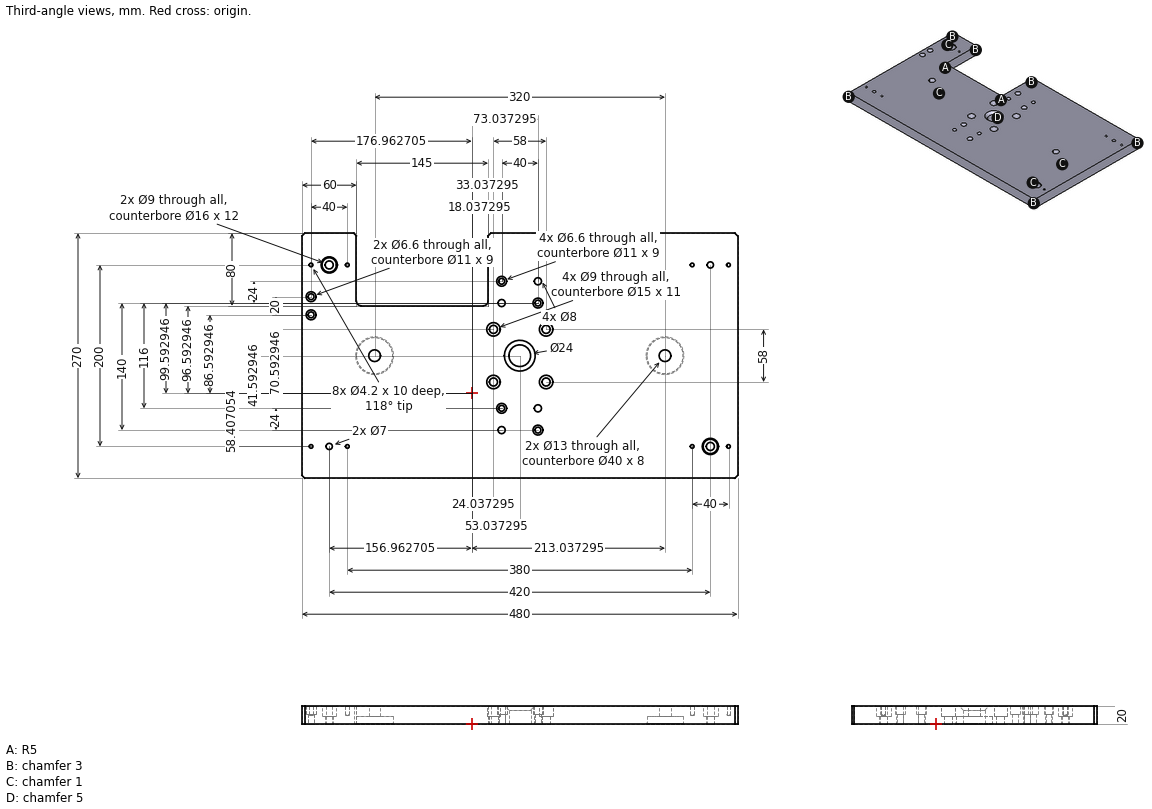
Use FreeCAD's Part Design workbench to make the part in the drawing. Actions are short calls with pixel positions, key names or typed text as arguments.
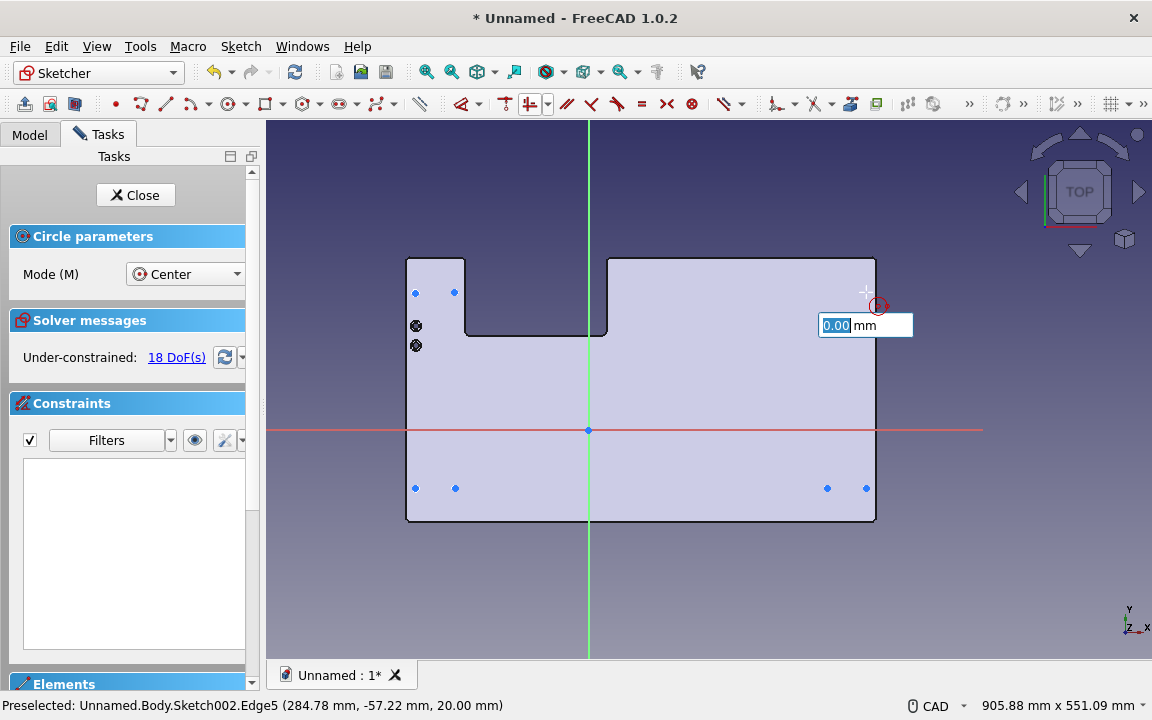
scroll(867, 290, up, 11)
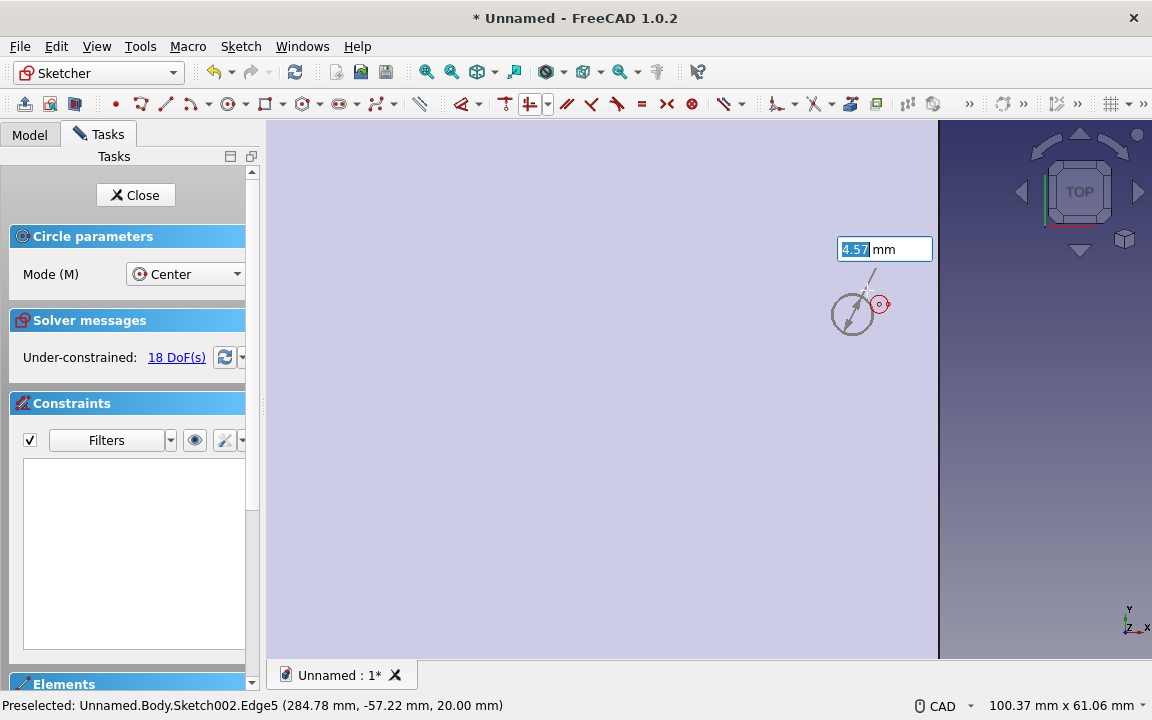
click(864, 290)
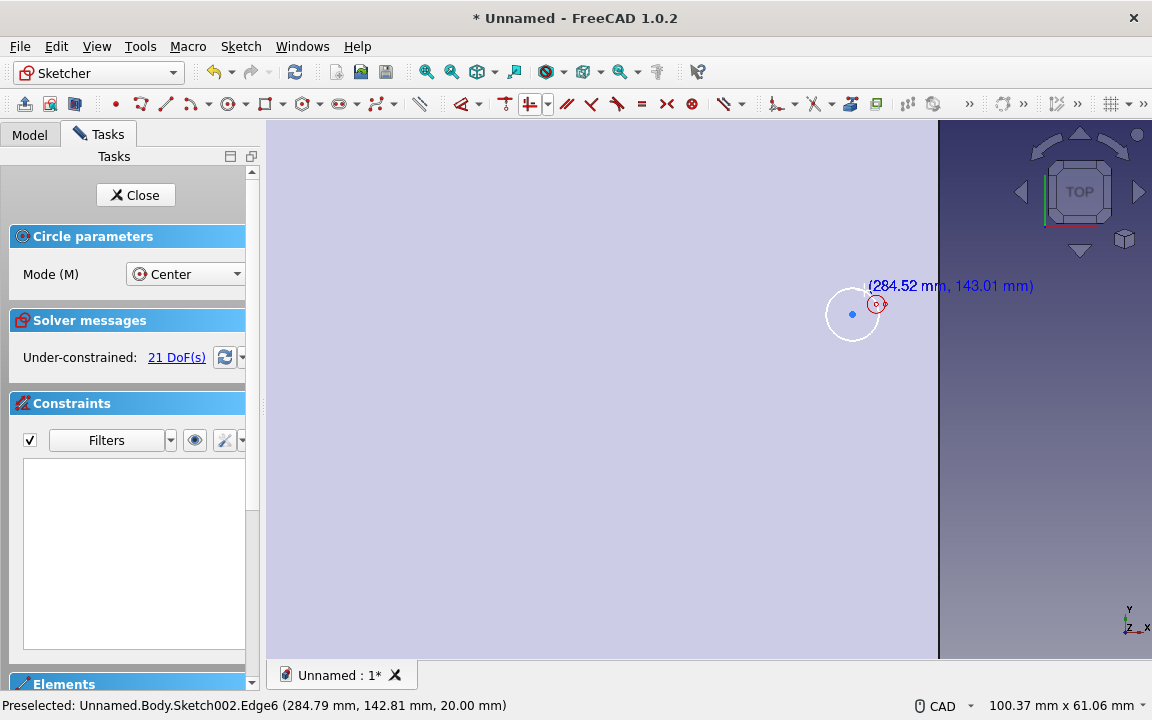
scroll(498, 304, up, 2)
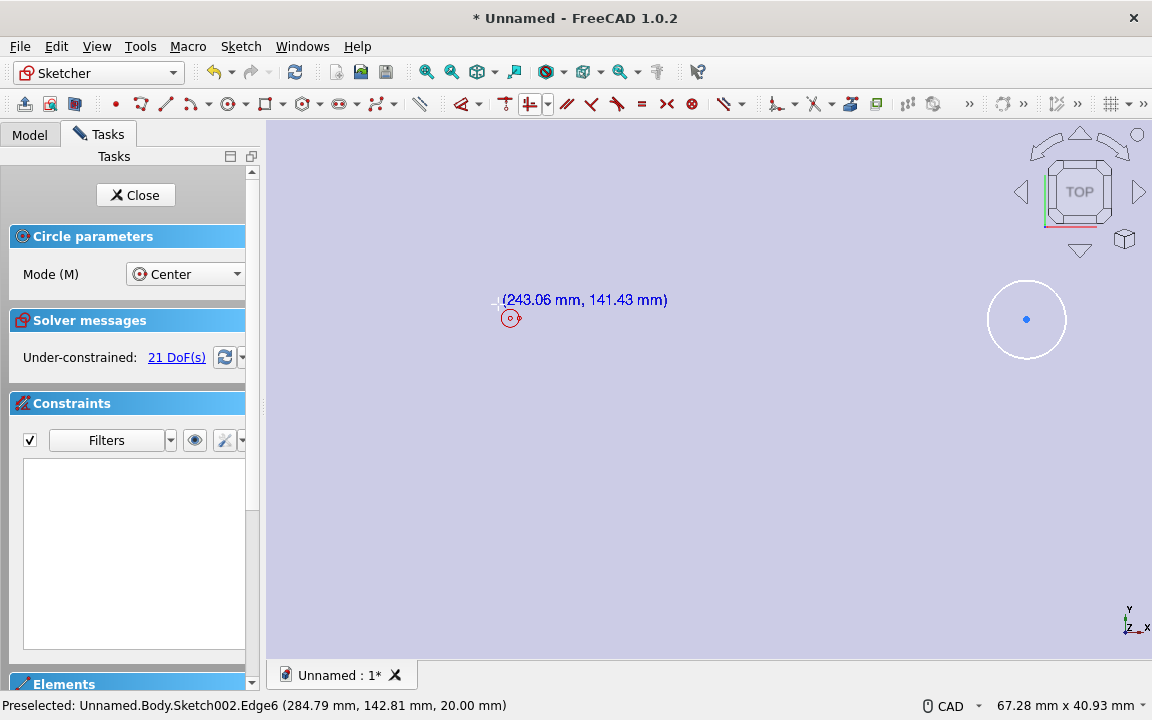
scroll(853, 291, down, 13)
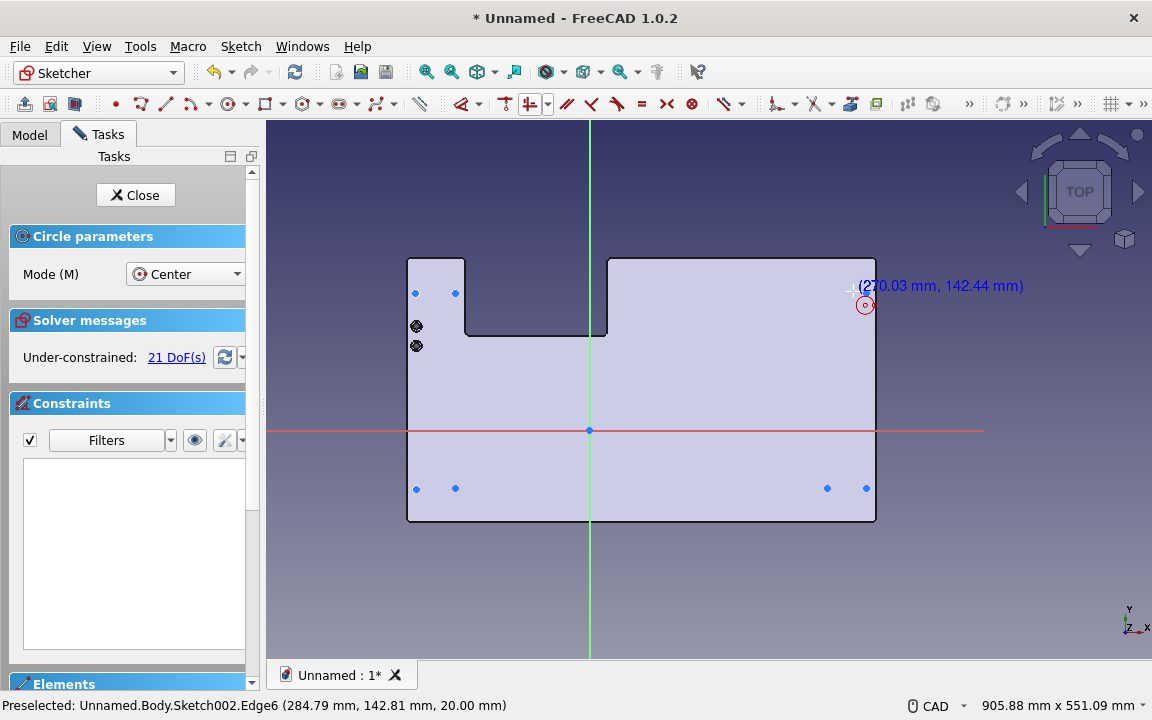
click(827, 292)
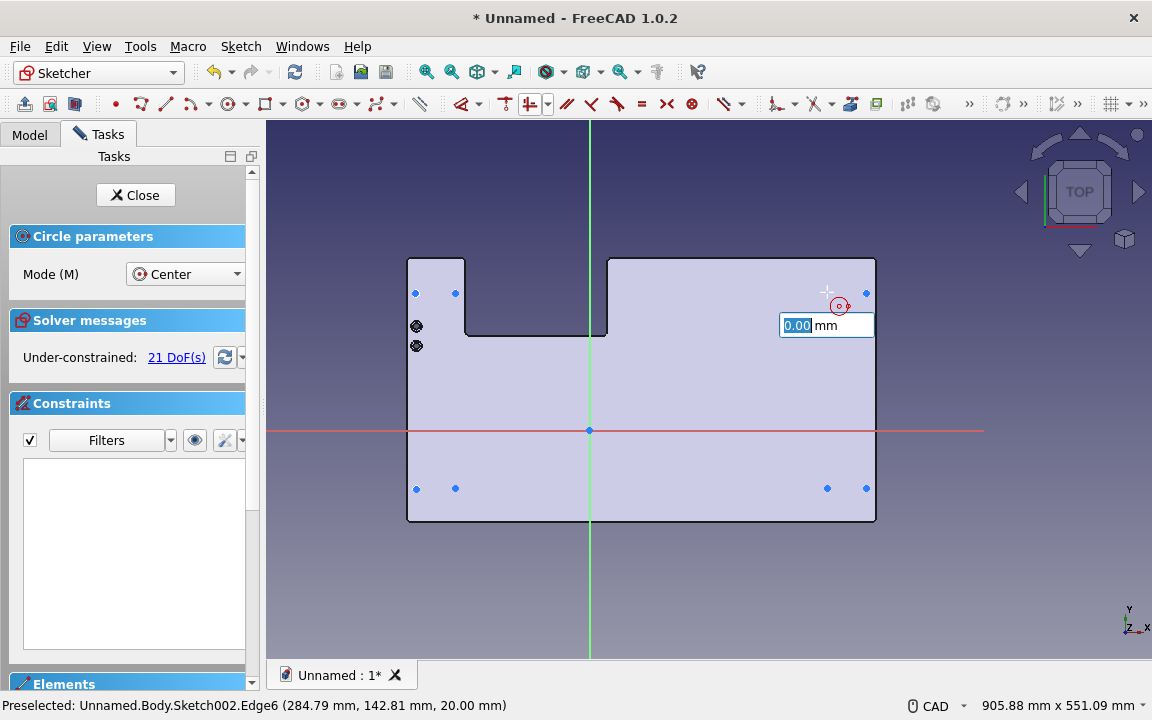
scroll(829, 291, up, 11)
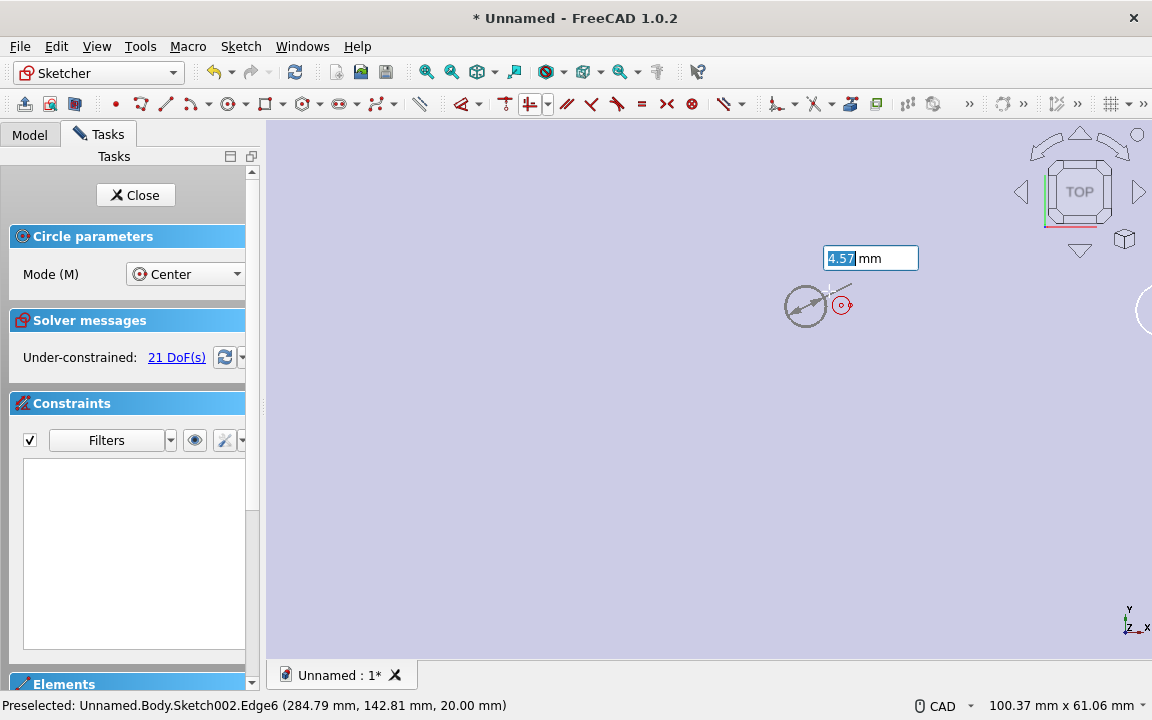
click(821, 286)
key(Escape)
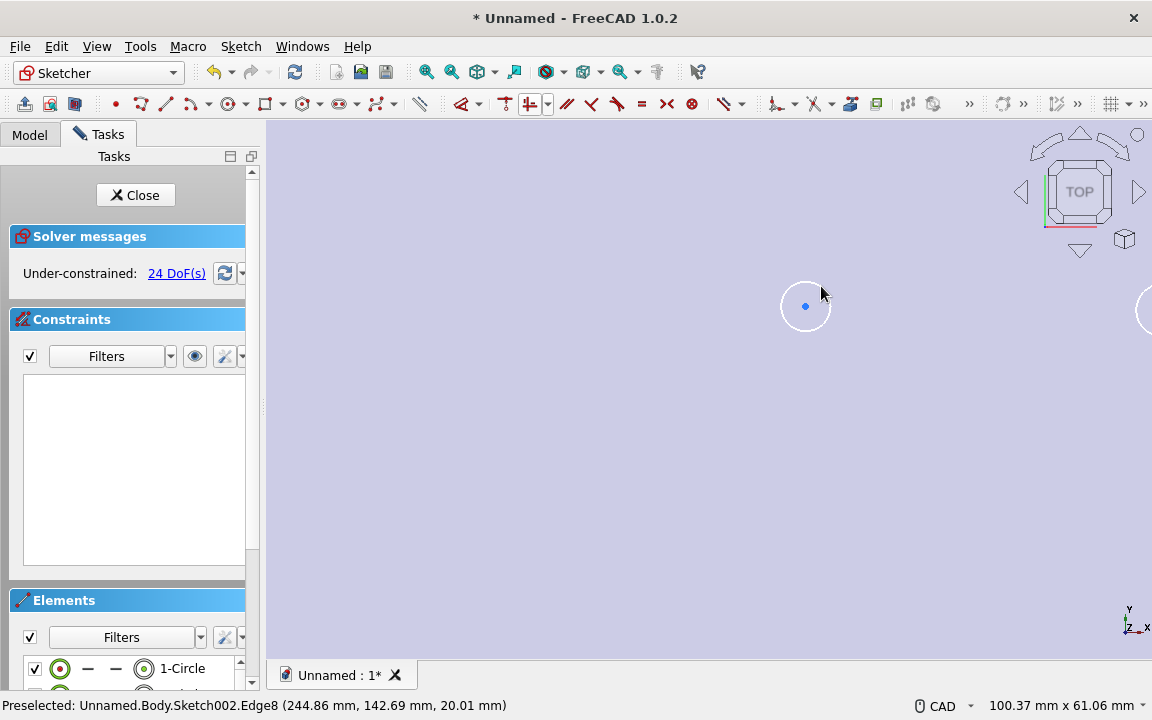
scroll(829, 291, down, 11)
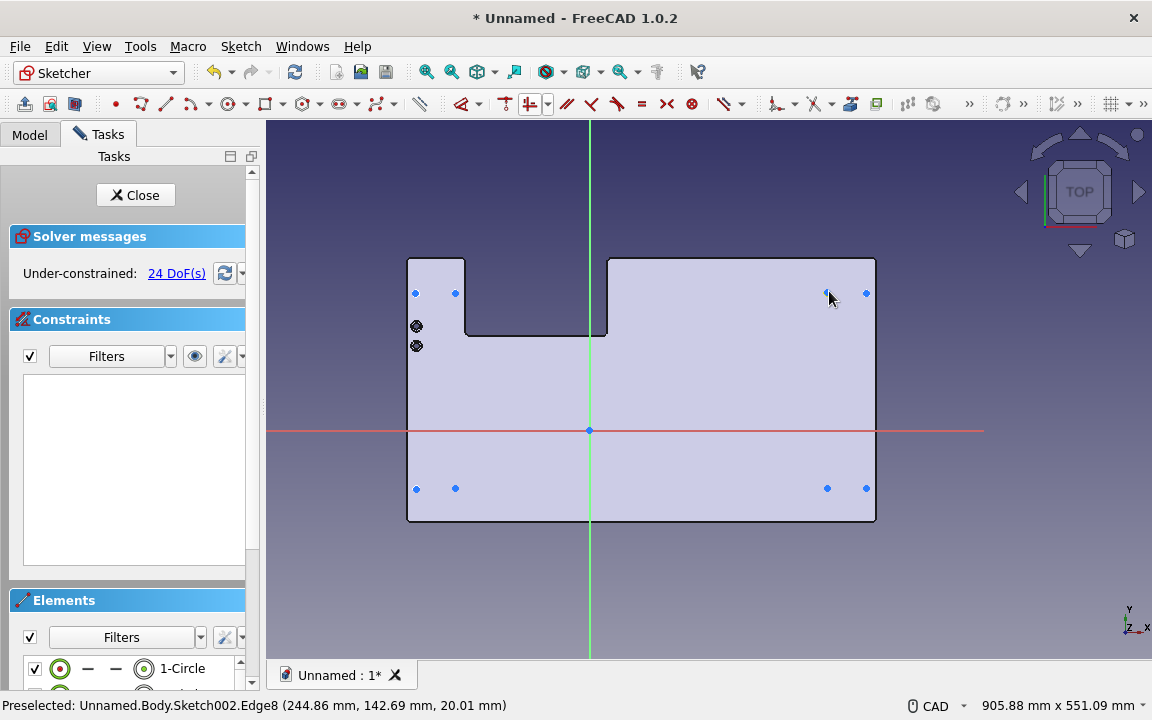
scroll(418, 291, up, 8)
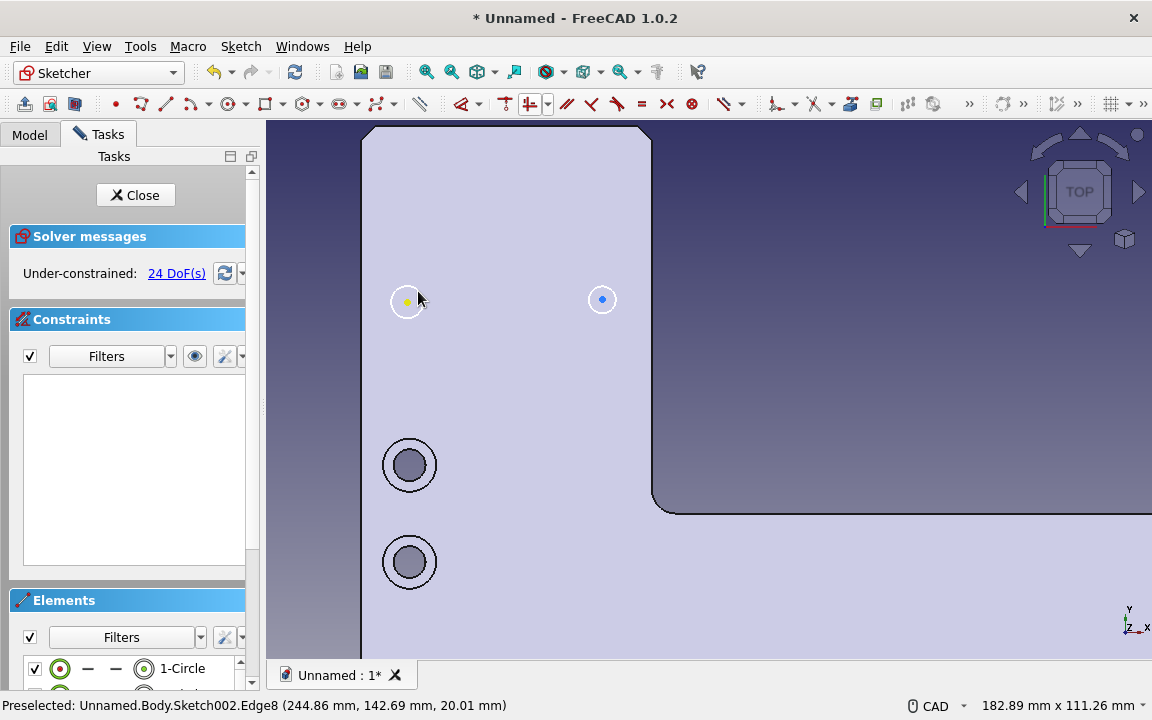
click(419, 291)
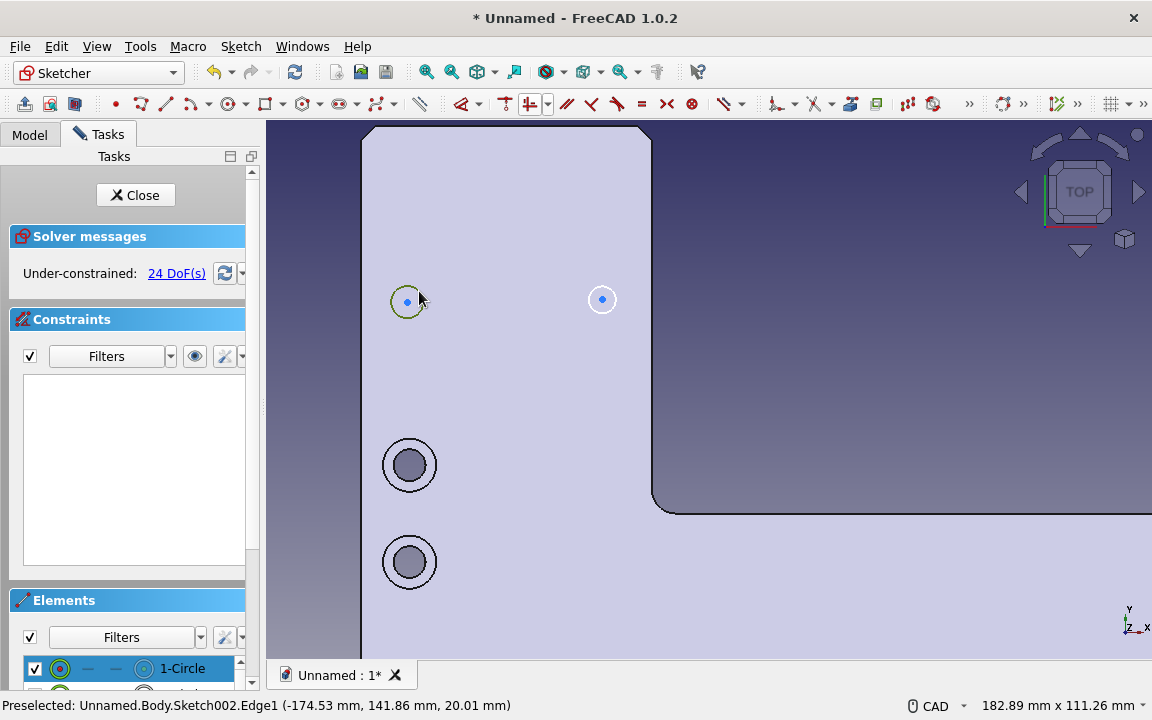
click(612, 290)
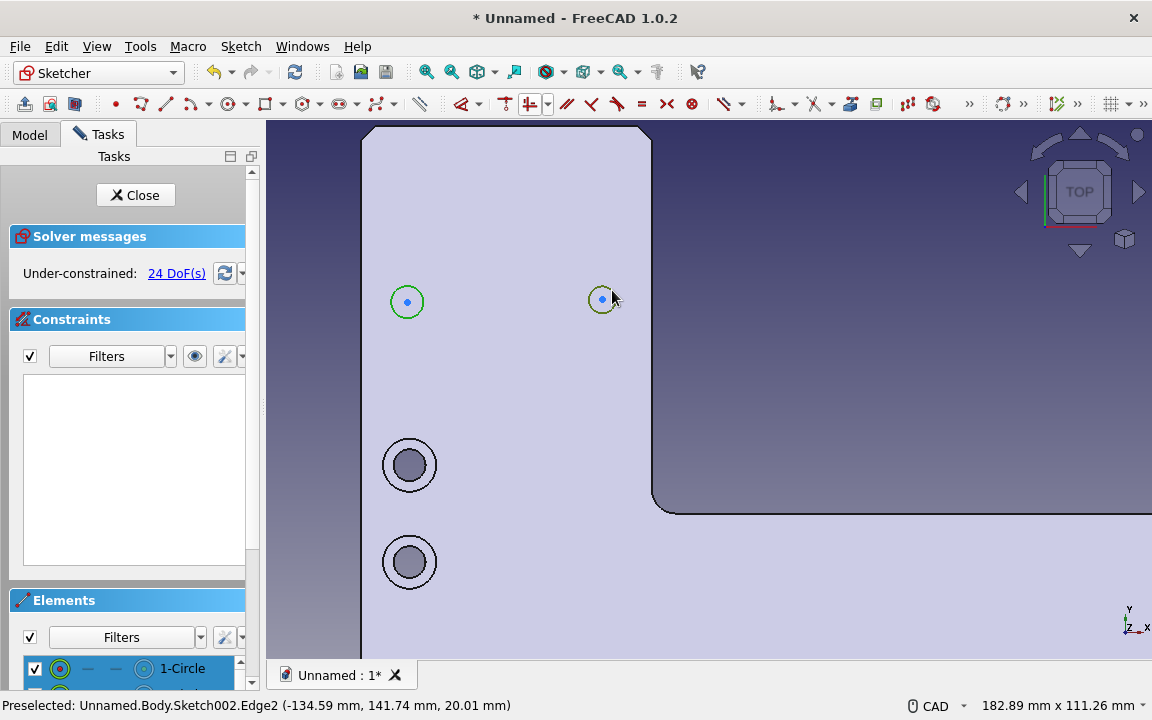
scroll(417, 291, down, 8)